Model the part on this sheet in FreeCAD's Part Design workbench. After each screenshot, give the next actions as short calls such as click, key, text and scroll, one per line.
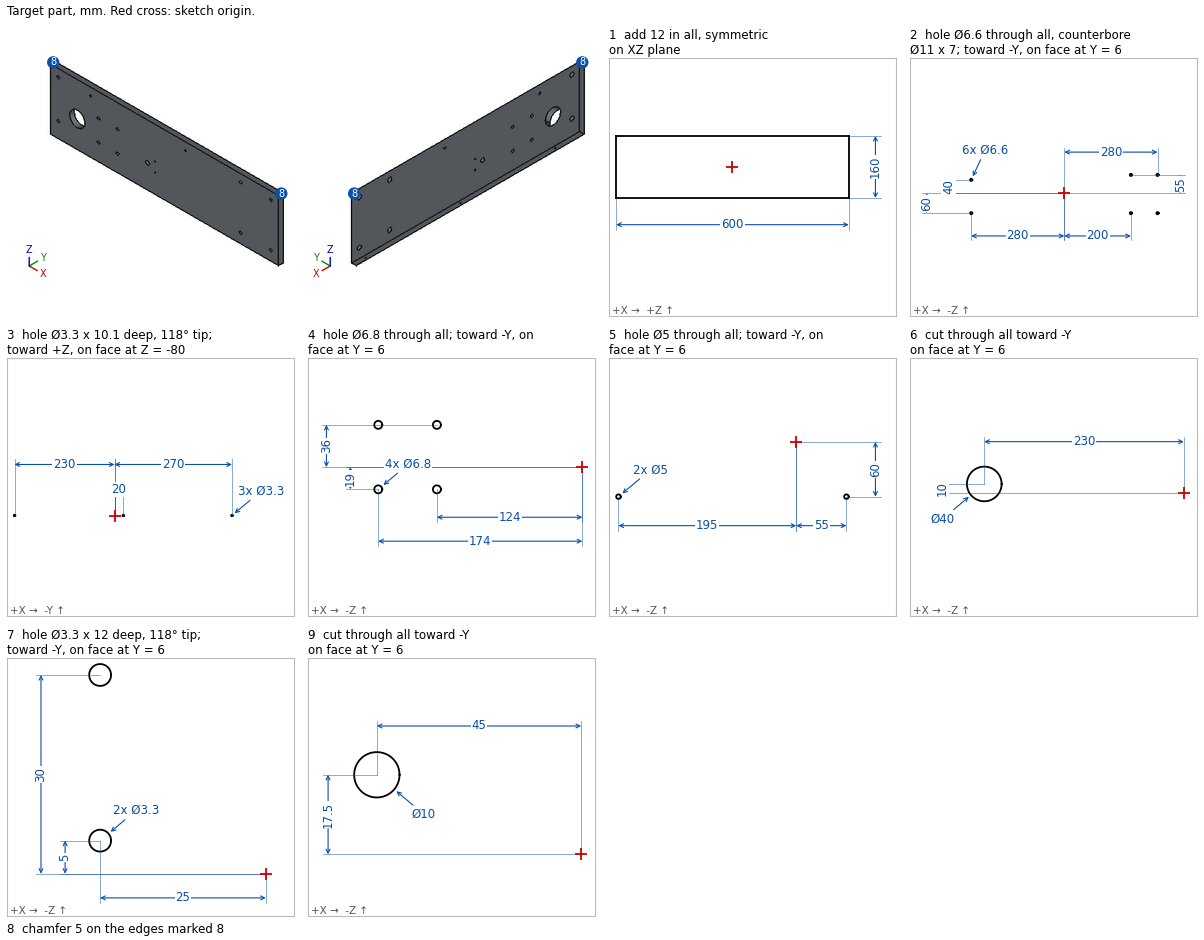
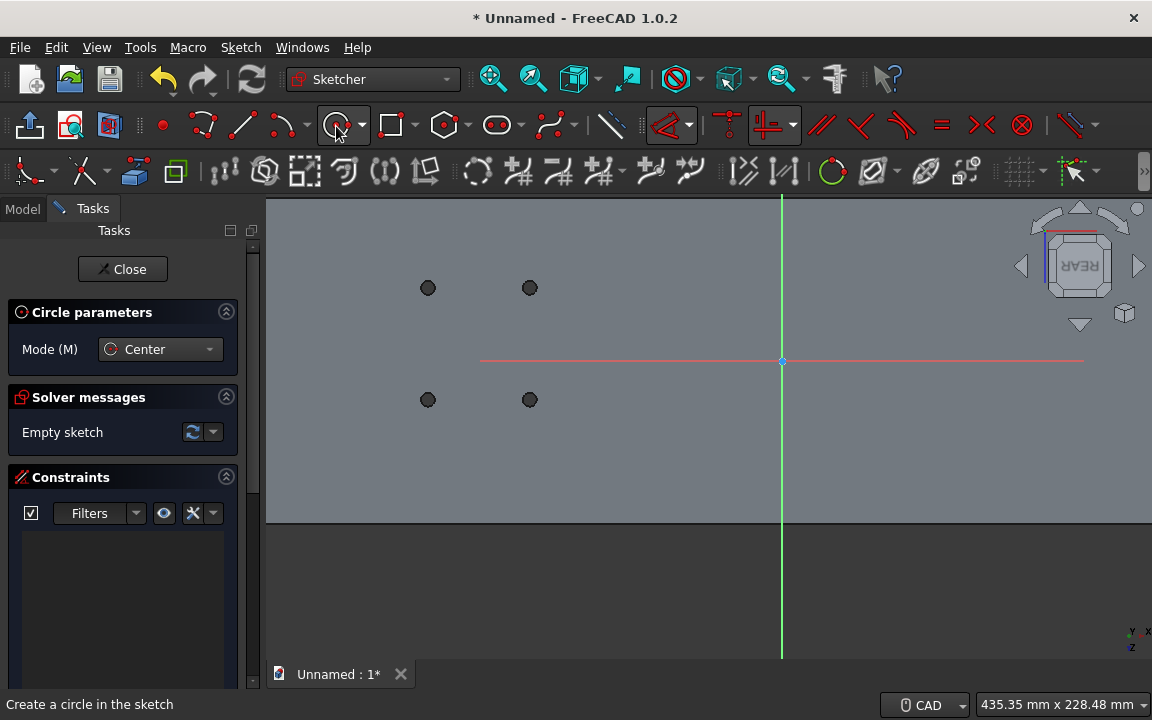
scroll(894, 483, up, 8)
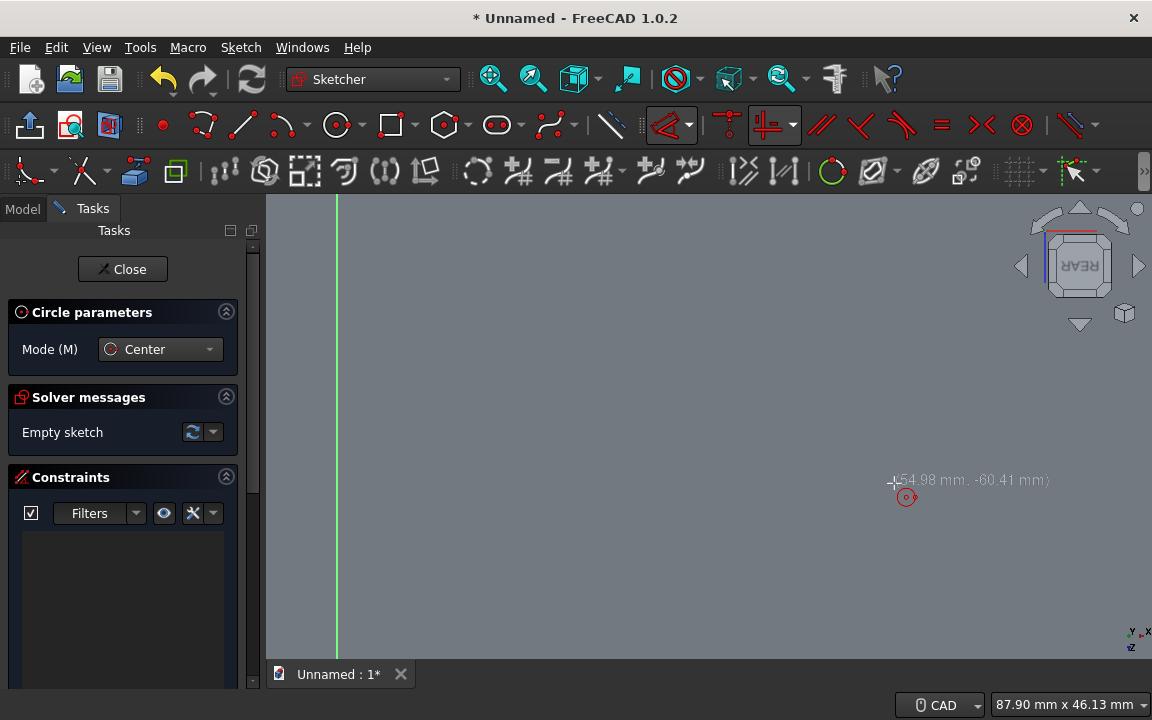
scroll(896, 486, down, 8)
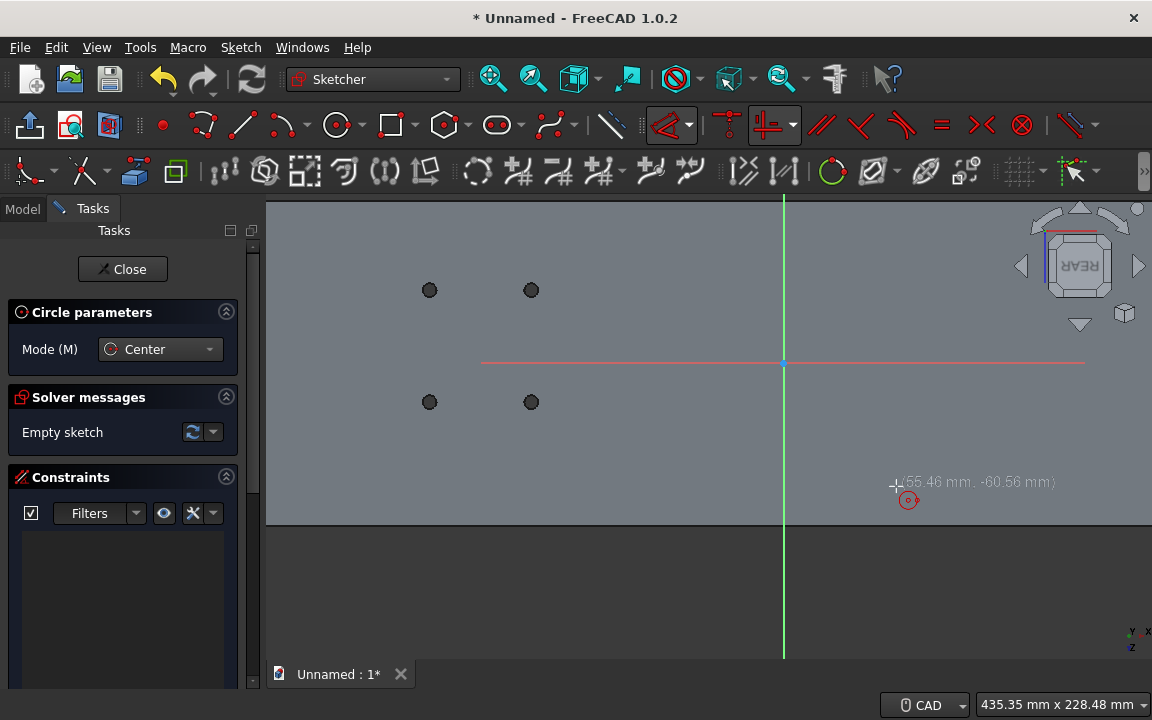
click(896, 486)
move(899, 482)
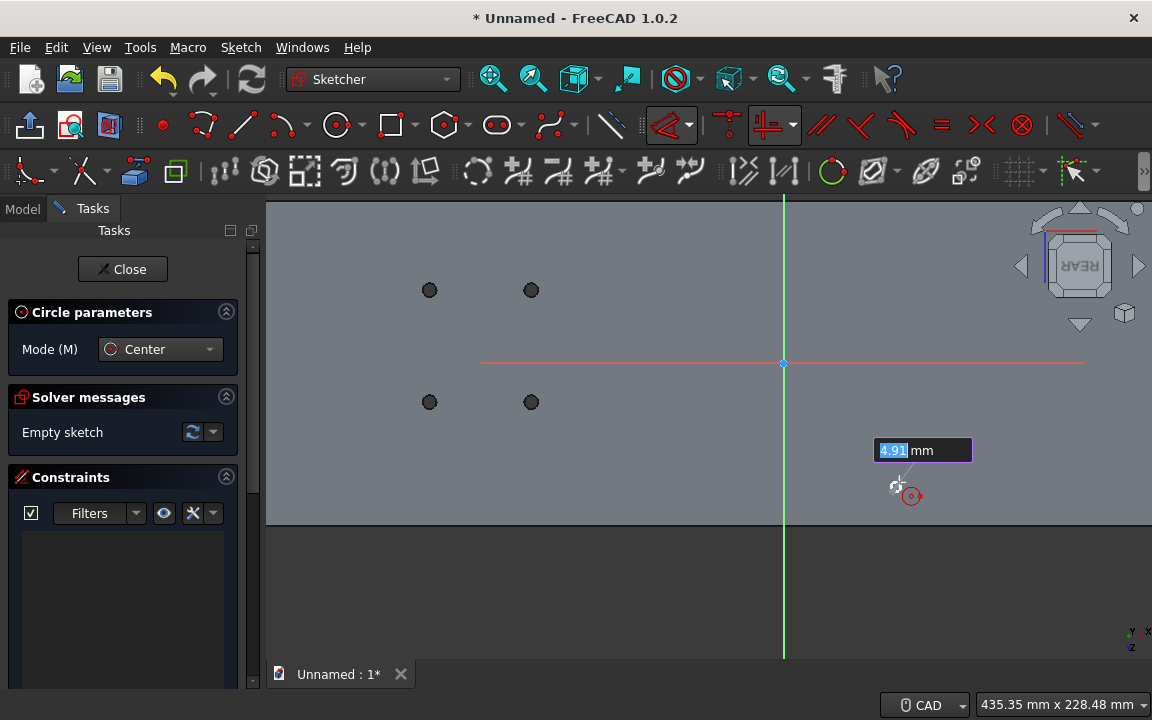
text(5)
key(Return)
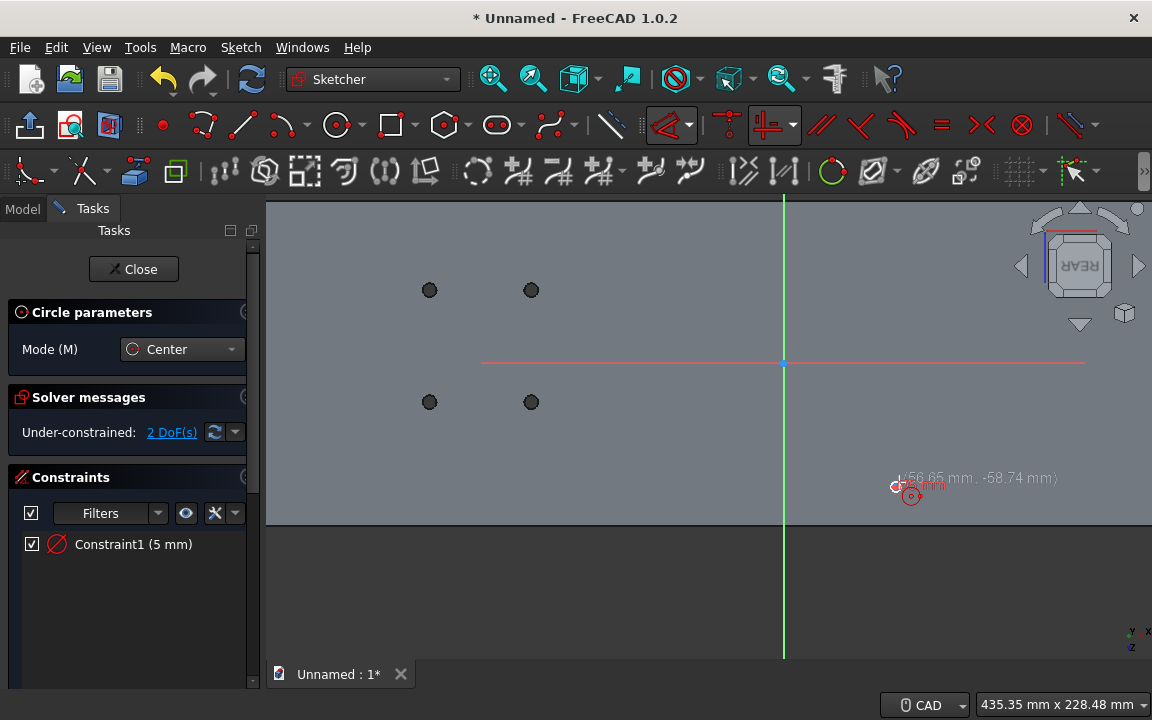
scroll(387, 486, up, 8)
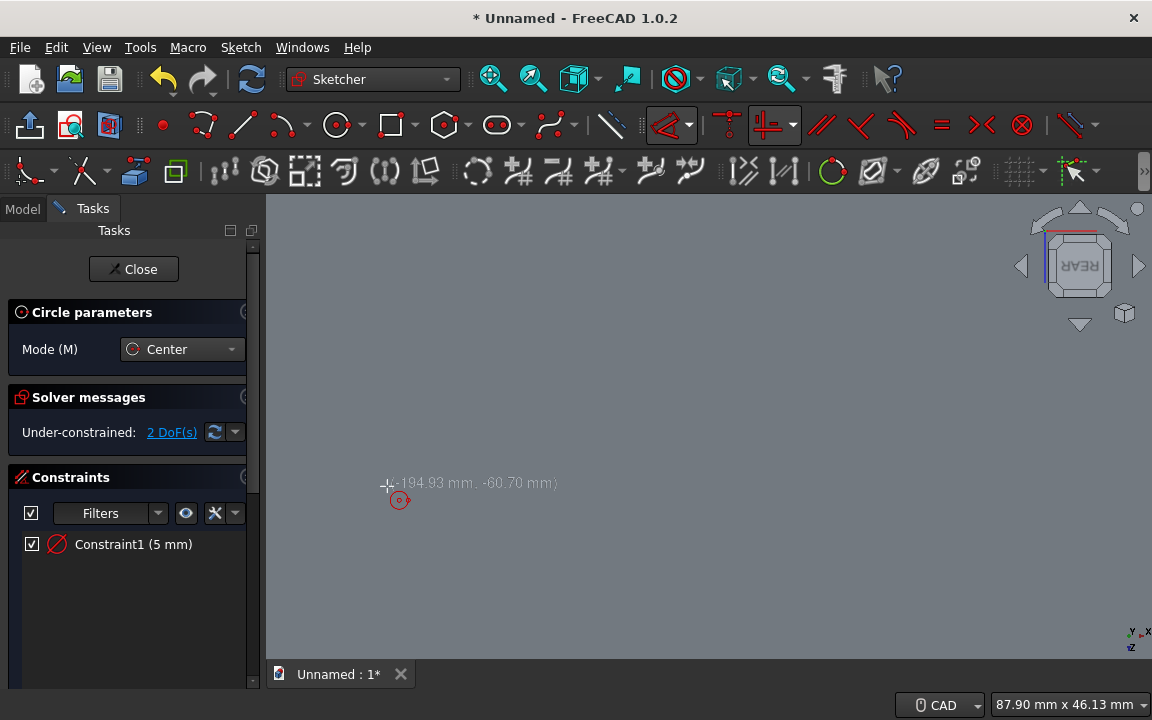
scroll(386, 486, down, 8)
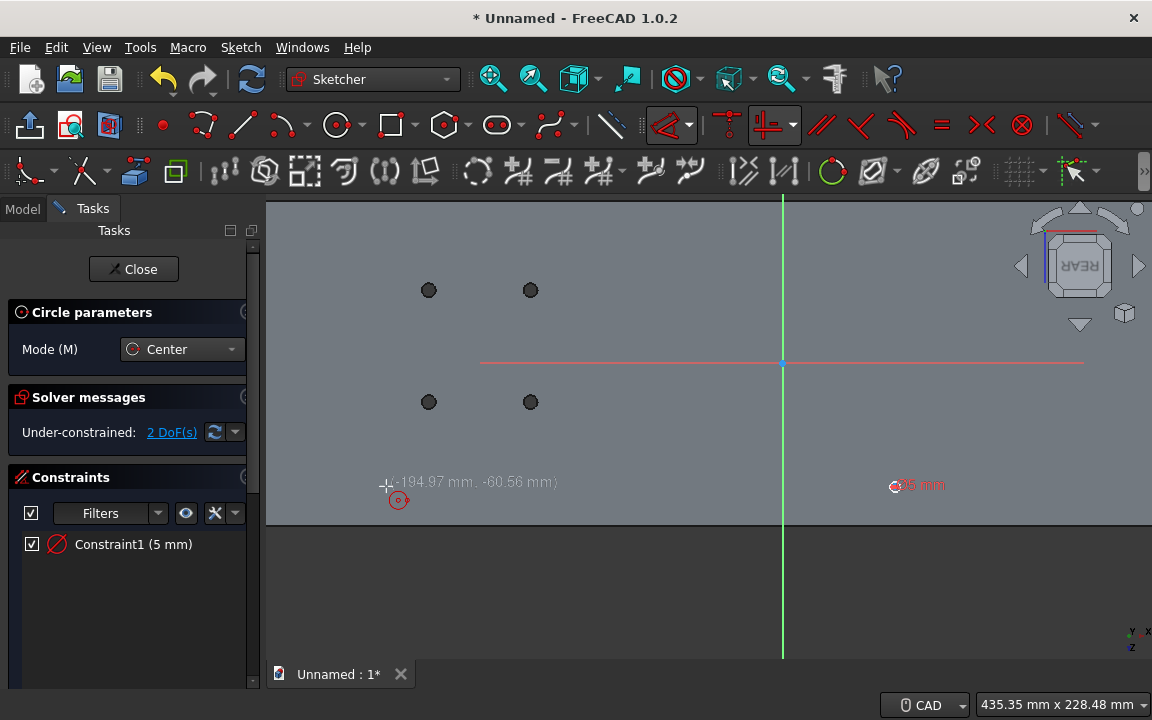
click(386, 486)
move(390, 482)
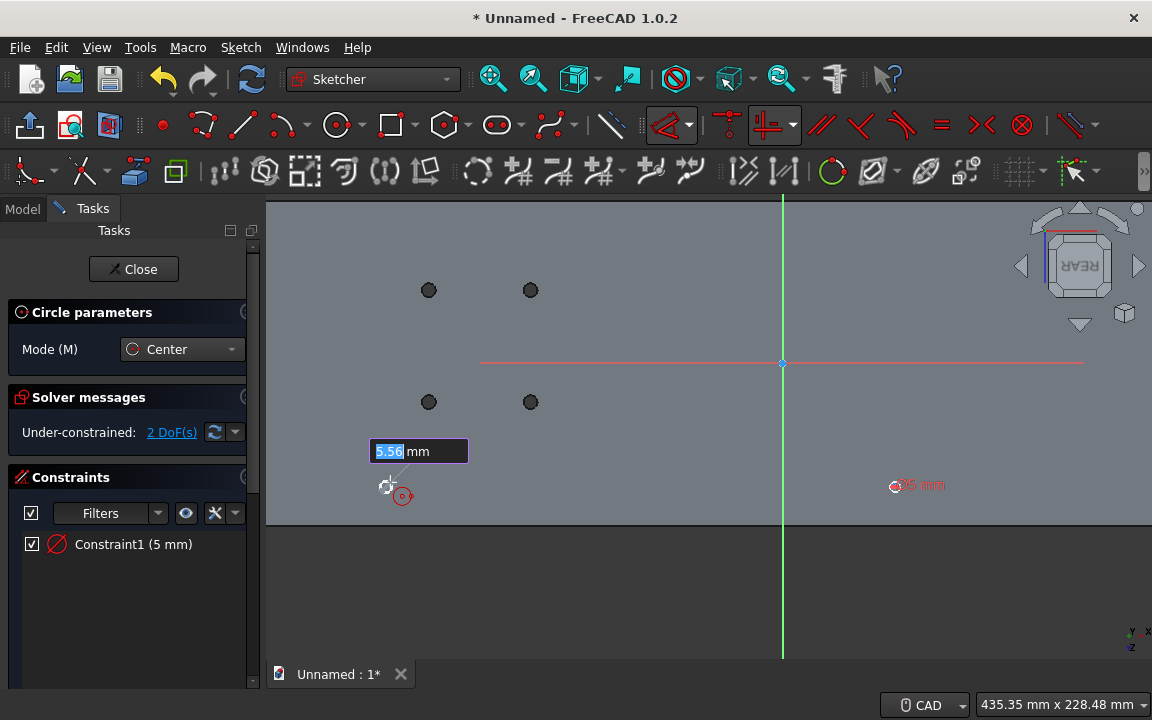
text(5)
key(Return)
key(Escape)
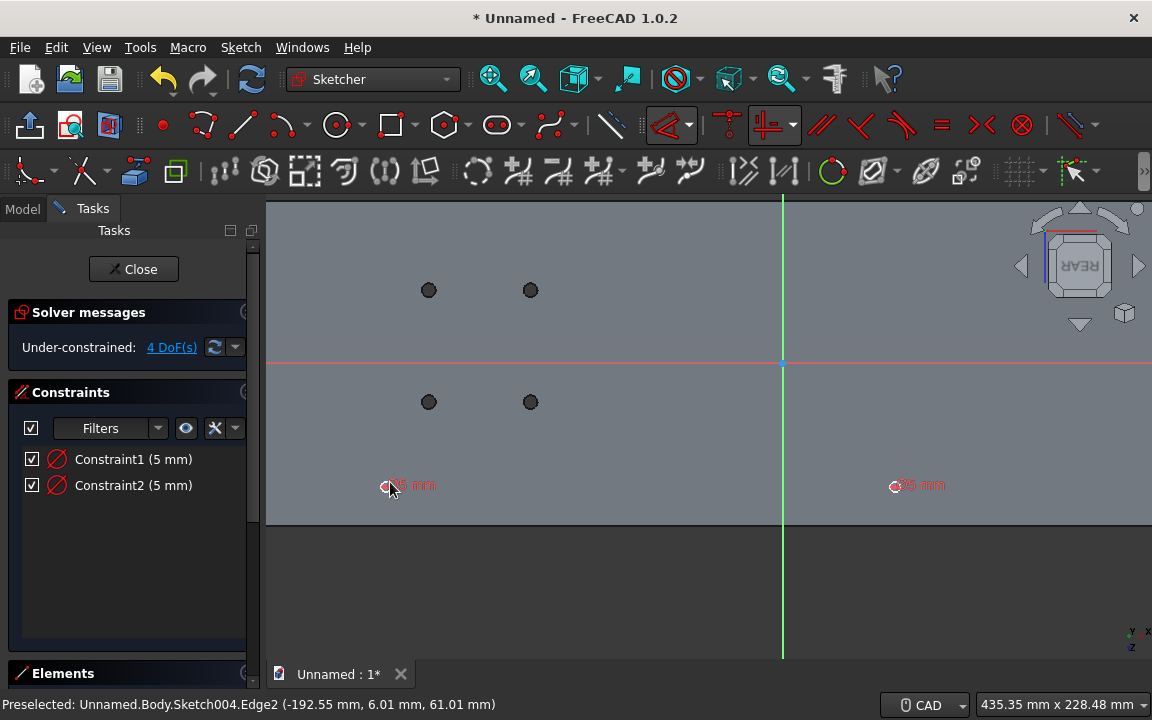
click(895, 487)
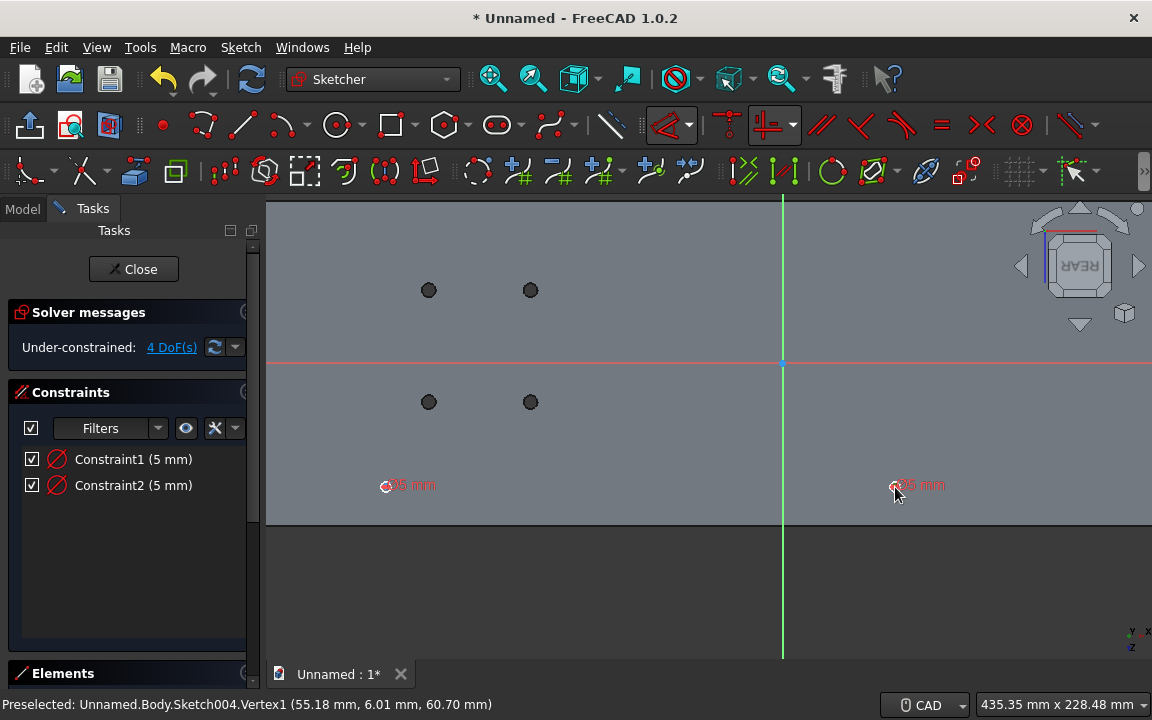
click(386, 487)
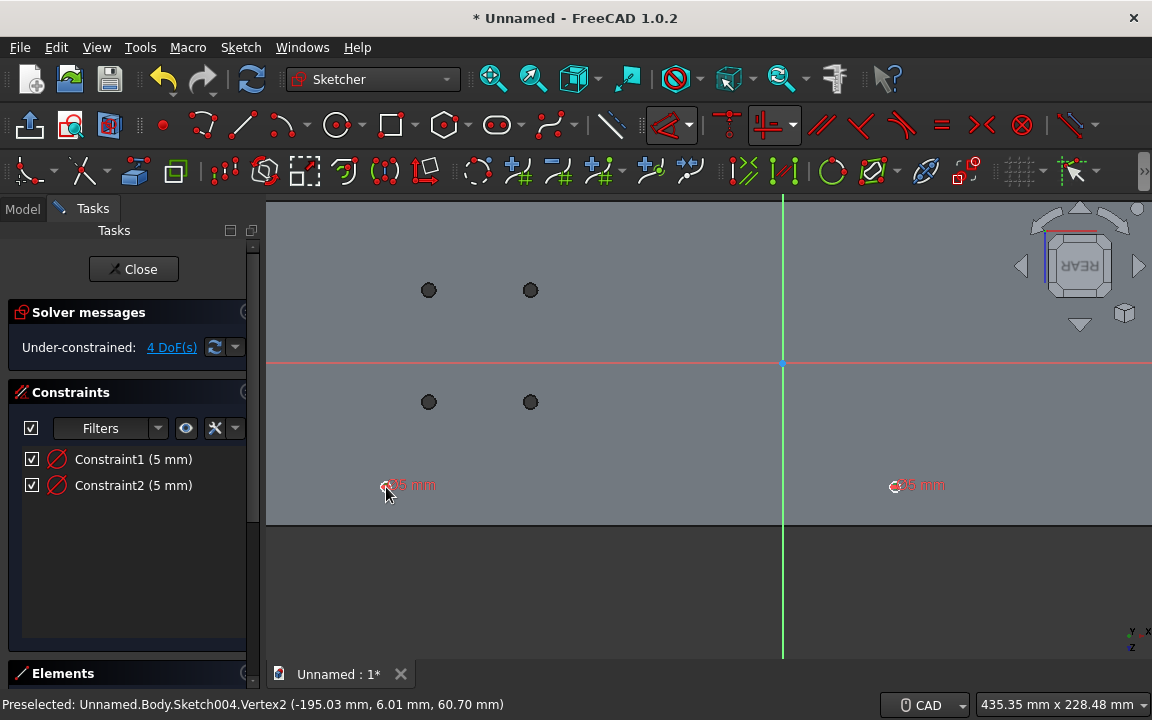
key(h)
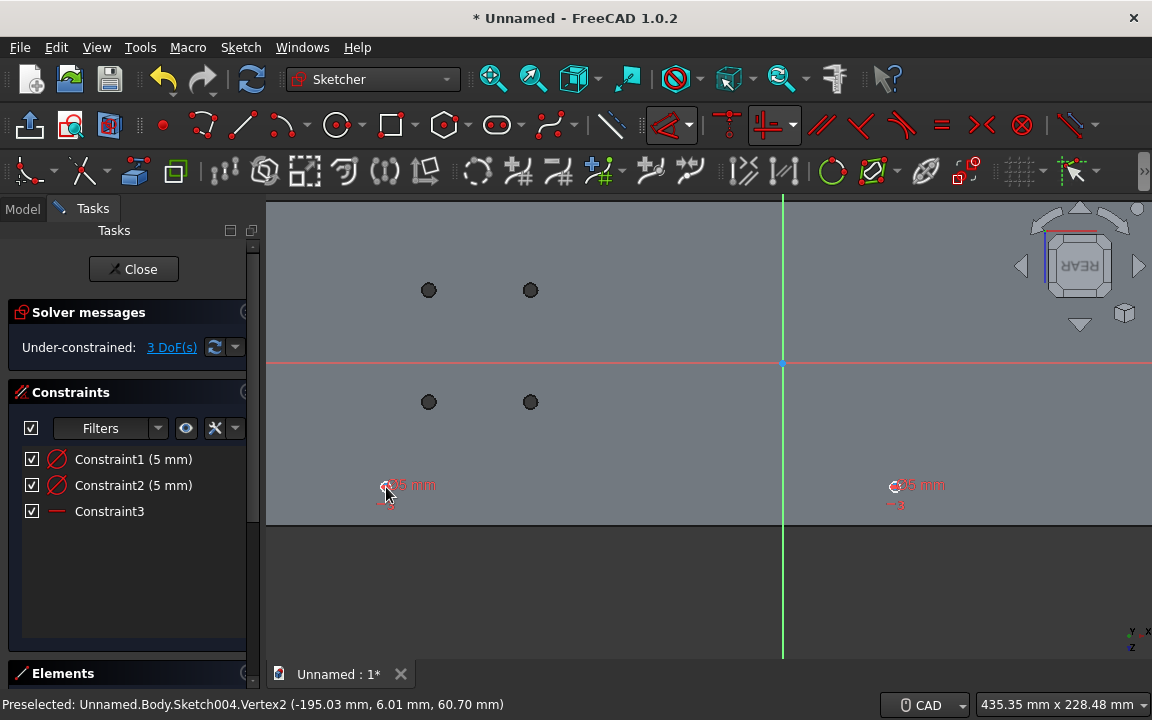
click(895, 487)